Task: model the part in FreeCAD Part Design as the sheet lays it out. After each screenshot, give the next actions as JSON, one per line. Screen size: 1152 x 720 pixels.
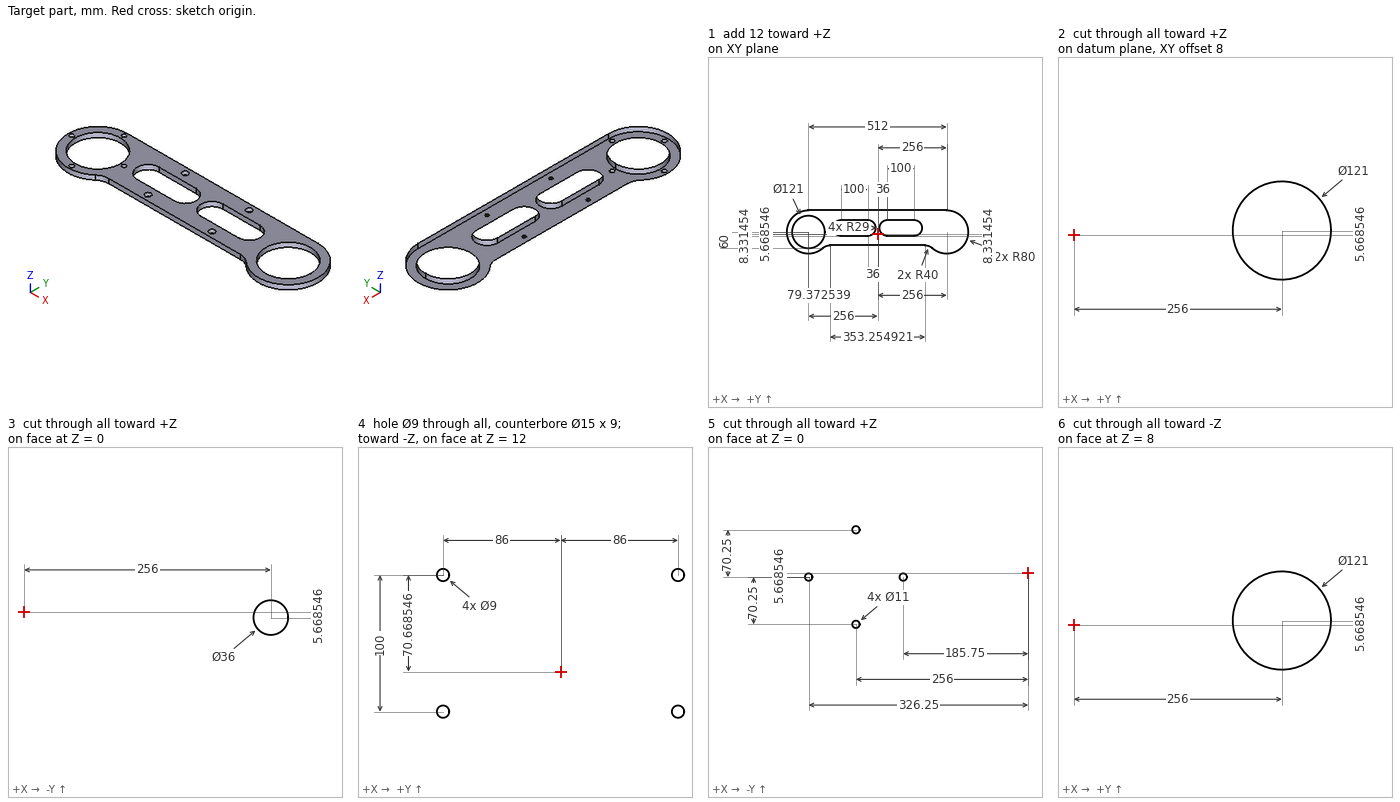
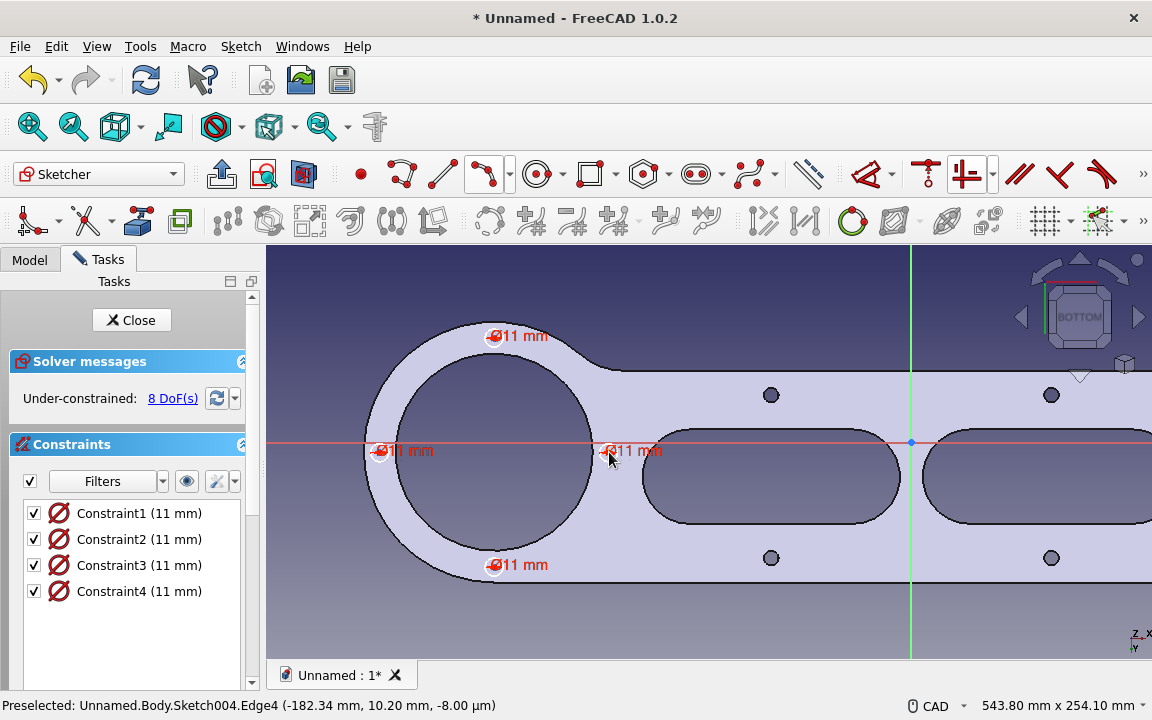
{"action": "left_click", "coordinate": [494, 567]}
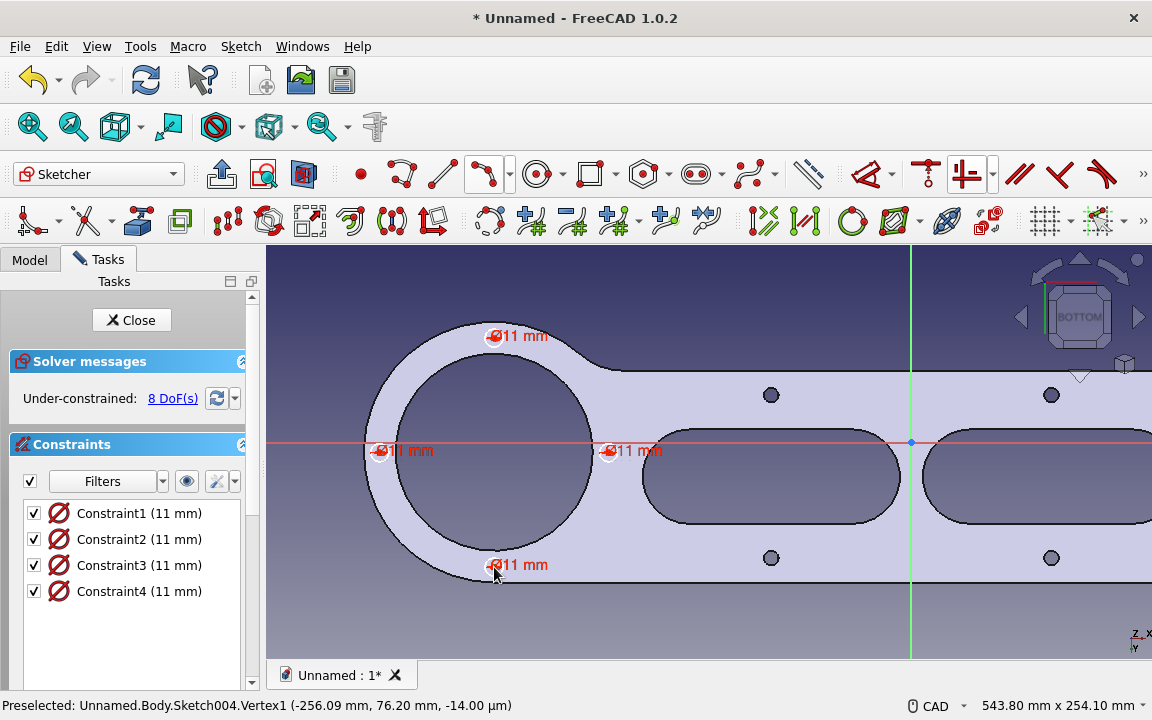
{"action": "left_click", "coordinate": [494, 338]}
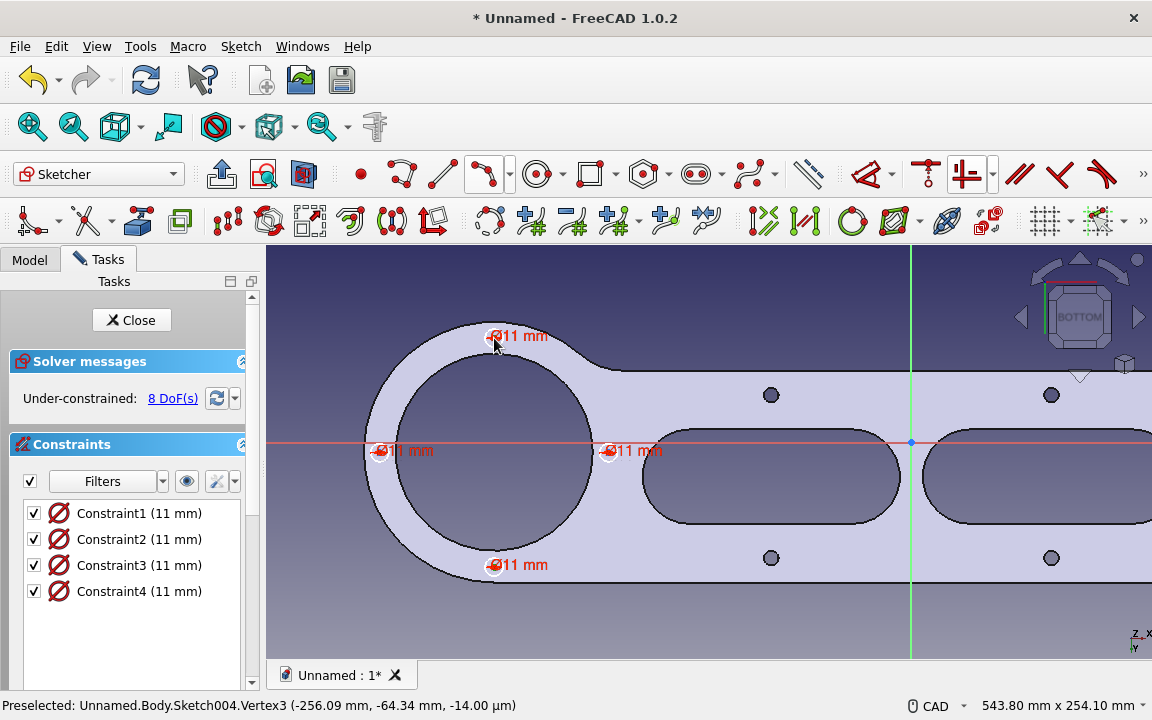
{"action": "left_click", "coordinate": [992, 174]}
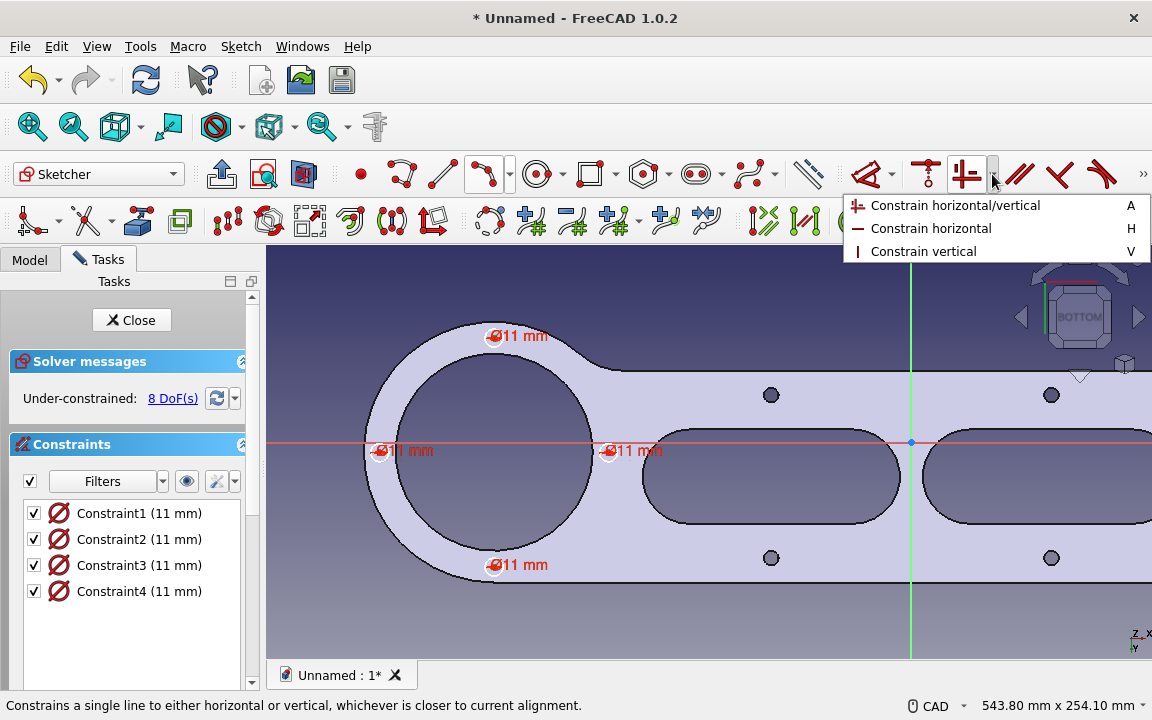
{"action": "left_click", "coordinate": [997, 252]}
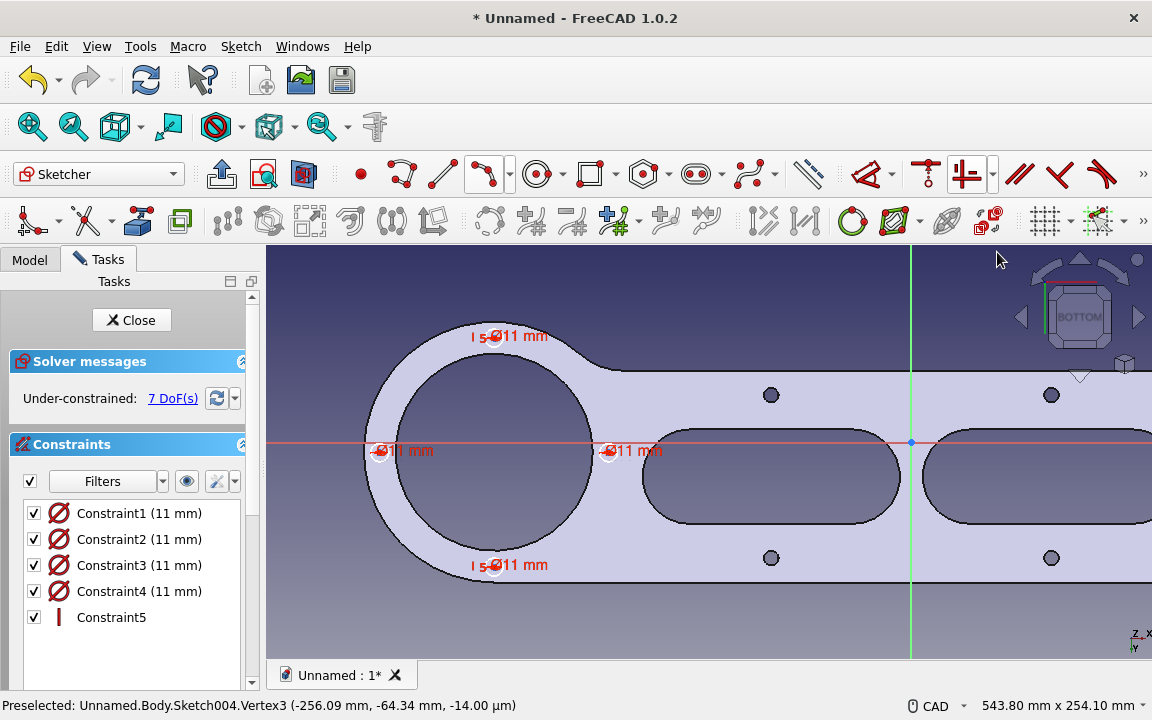
{"action": "left_click", "coordinate": [380, 453]}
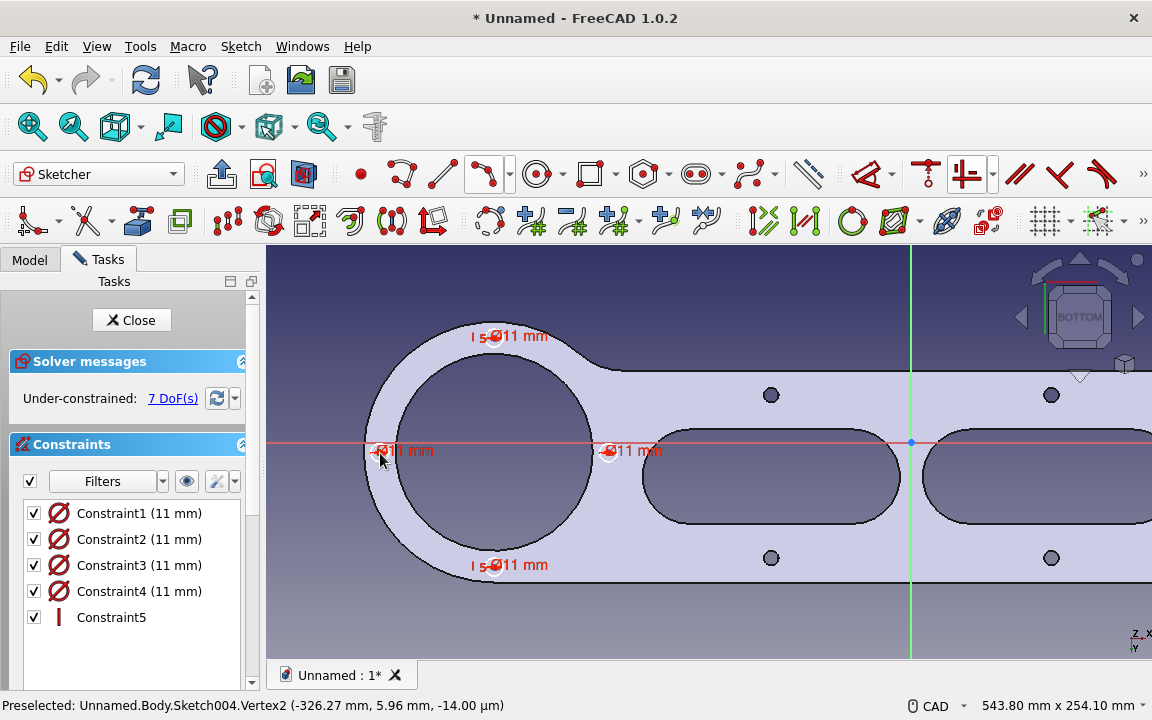
{"action": "left_click", "coordinate": [609, 453]}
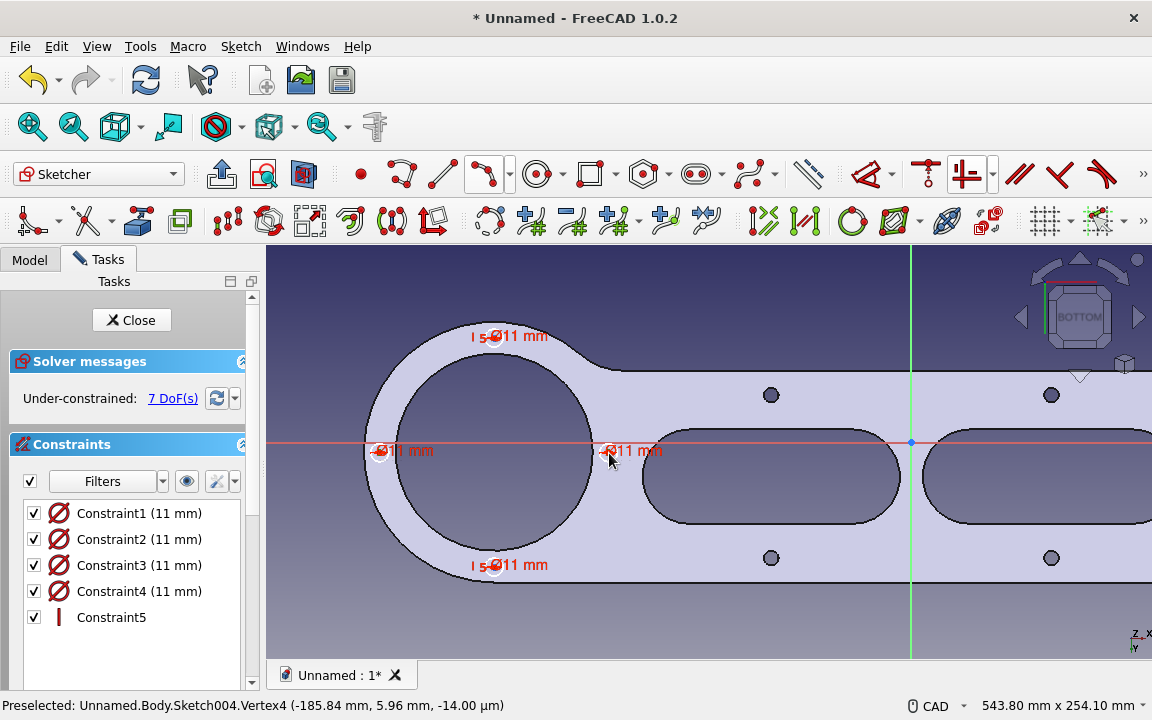
{"action": "left_click", "coordinate": [992, 174]}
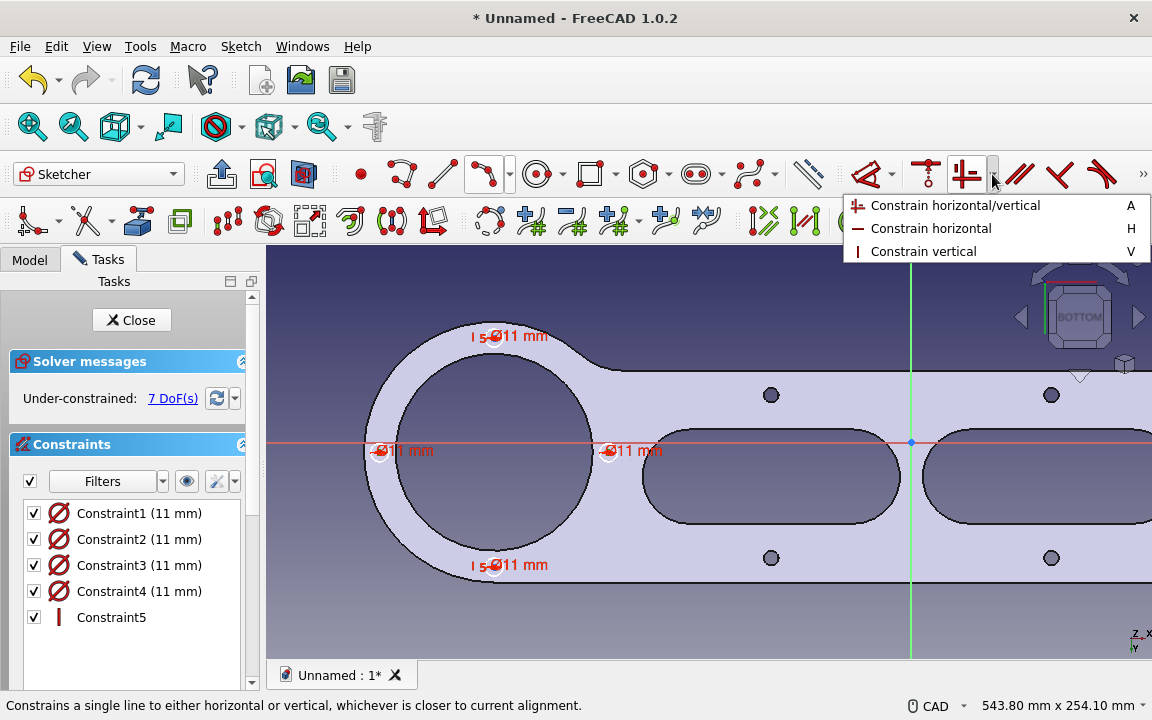
{"action": "left_click", "coordinate": [997, 228]}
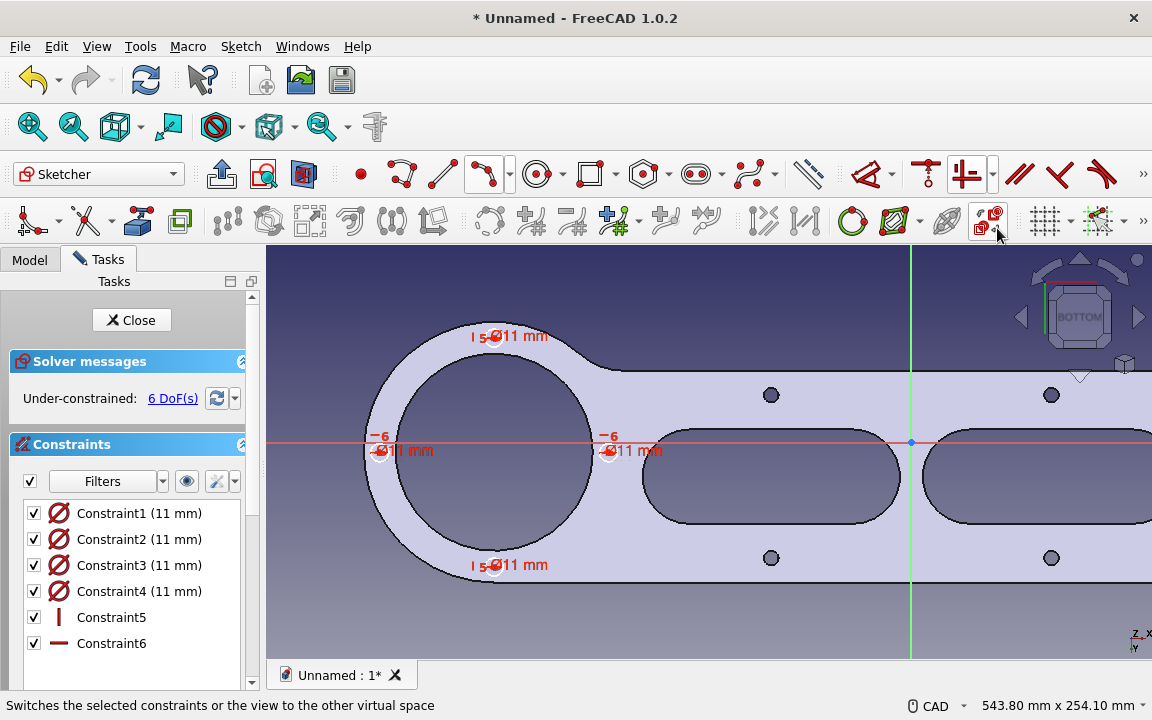
{"action": "left_click", "coordinate": [866, 174]}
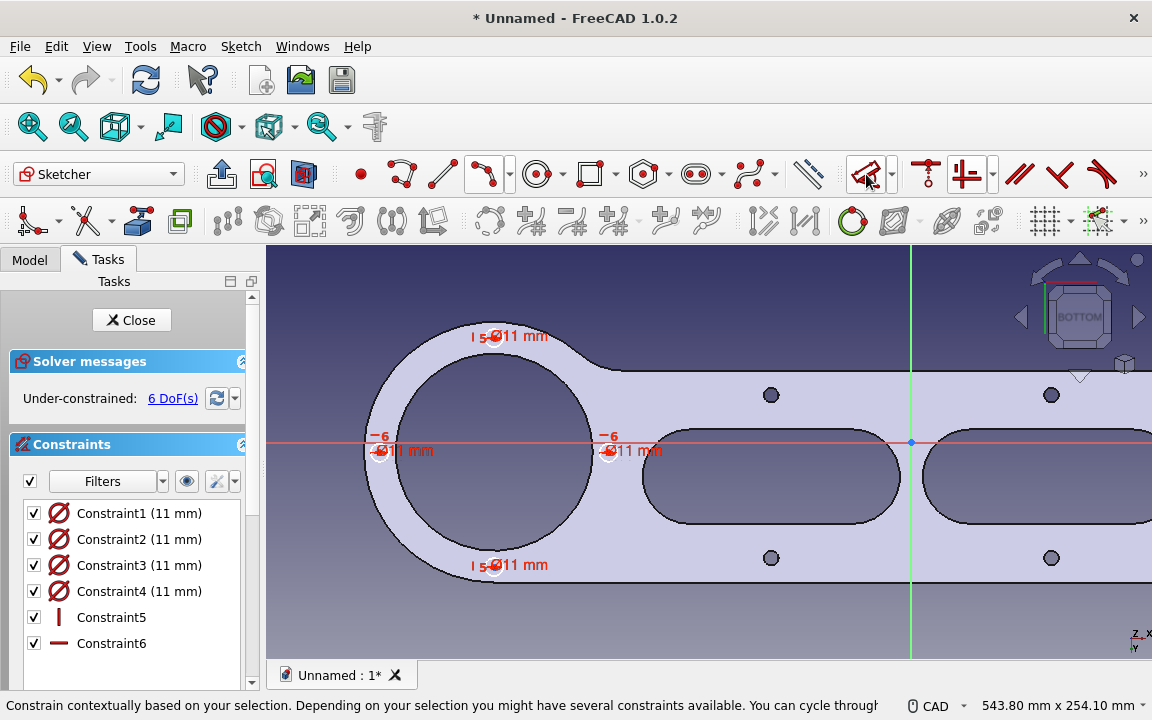
{"action": "left_click", "coordinate": [494, 567]}
{"action": "left_click", "coordinate": [703, 601]}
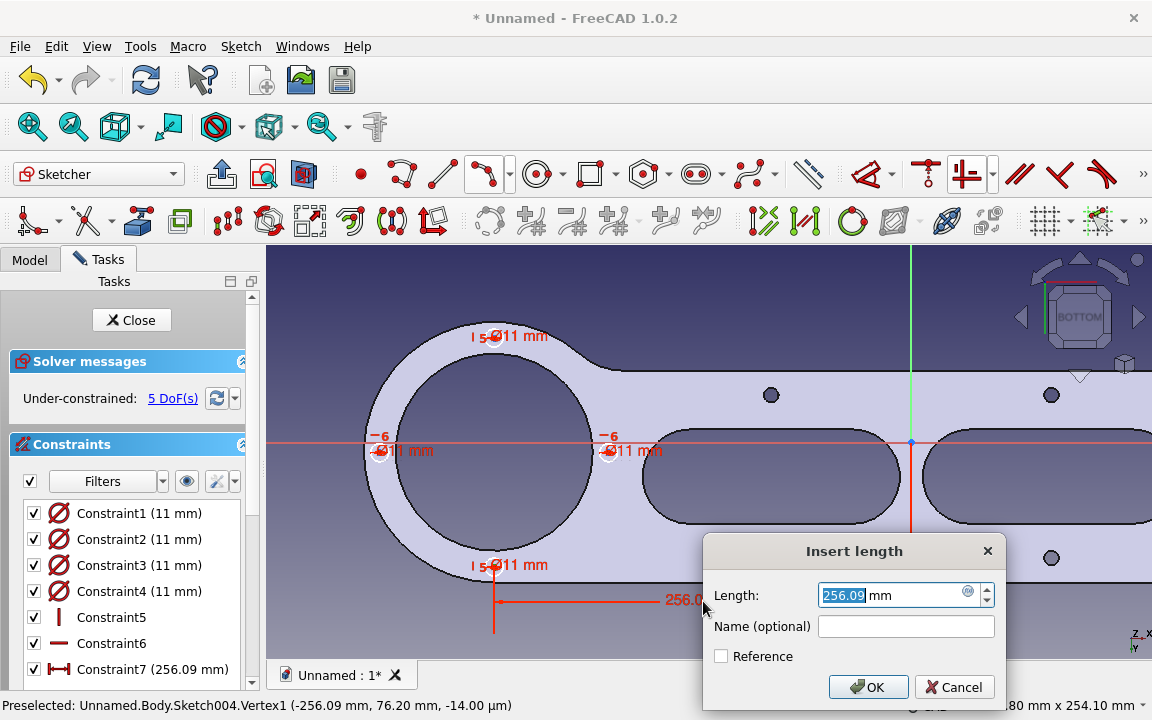
{"action": "type", "text": "256"}
{"action": "key", "text": "Return"}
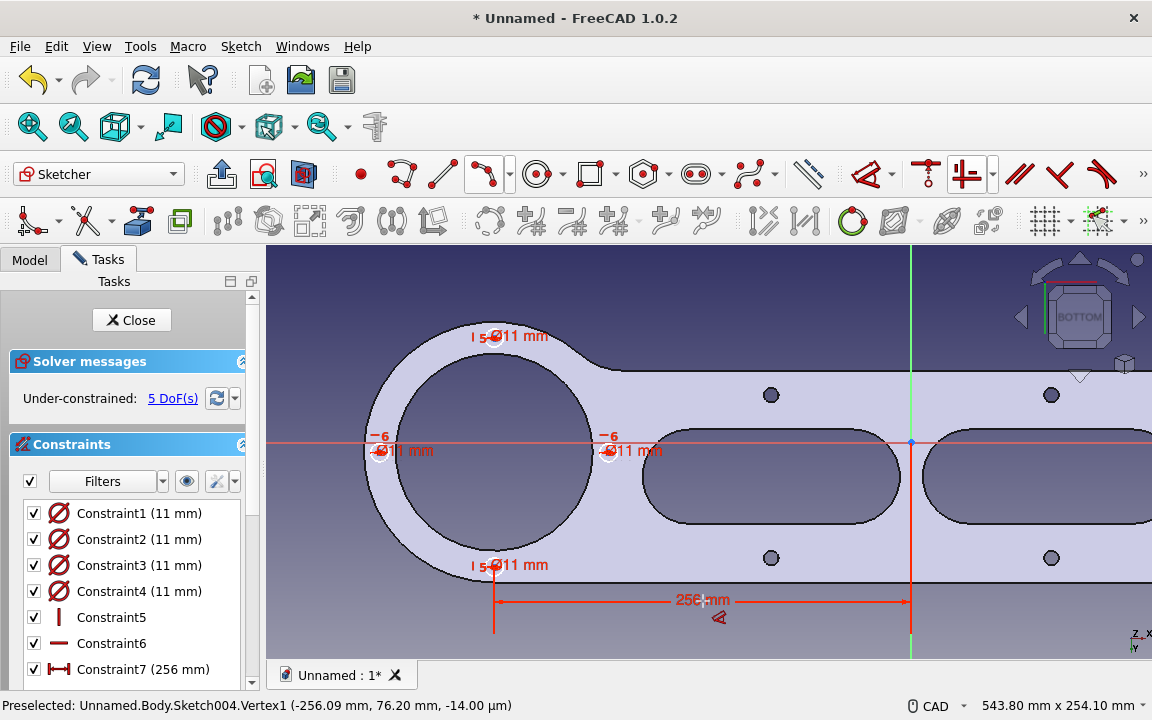
{"action": "left_click", "coordinate": [380, 453]}
{"action": "left_click", "coordinate": [646, 409]}